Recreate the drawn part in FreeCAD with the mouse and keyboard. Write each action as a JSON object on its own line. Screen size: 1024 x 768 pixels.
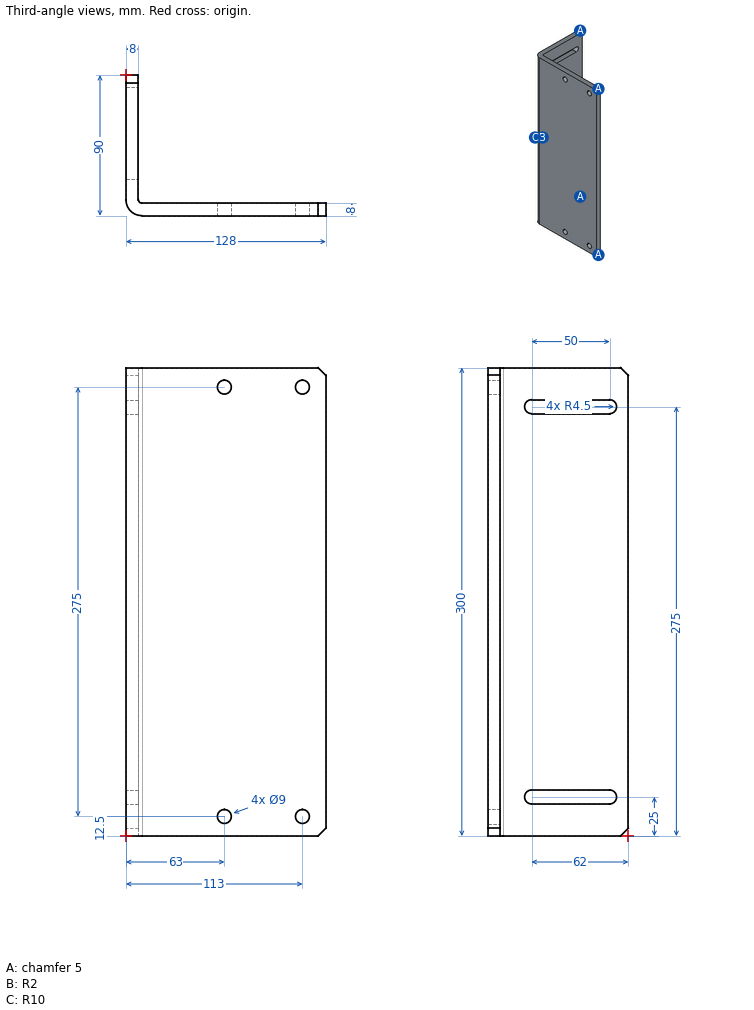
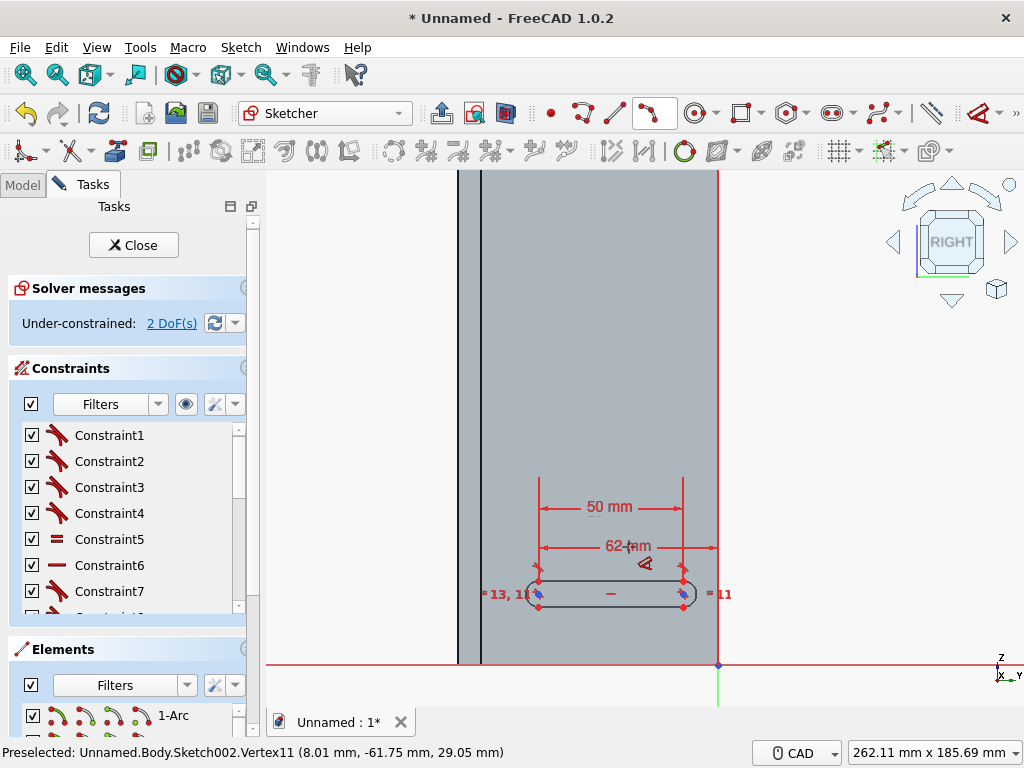
{"action": "left_click", "coordinate": [539, 594]}
{"action": "left_click", "coordinate": [752, 630]}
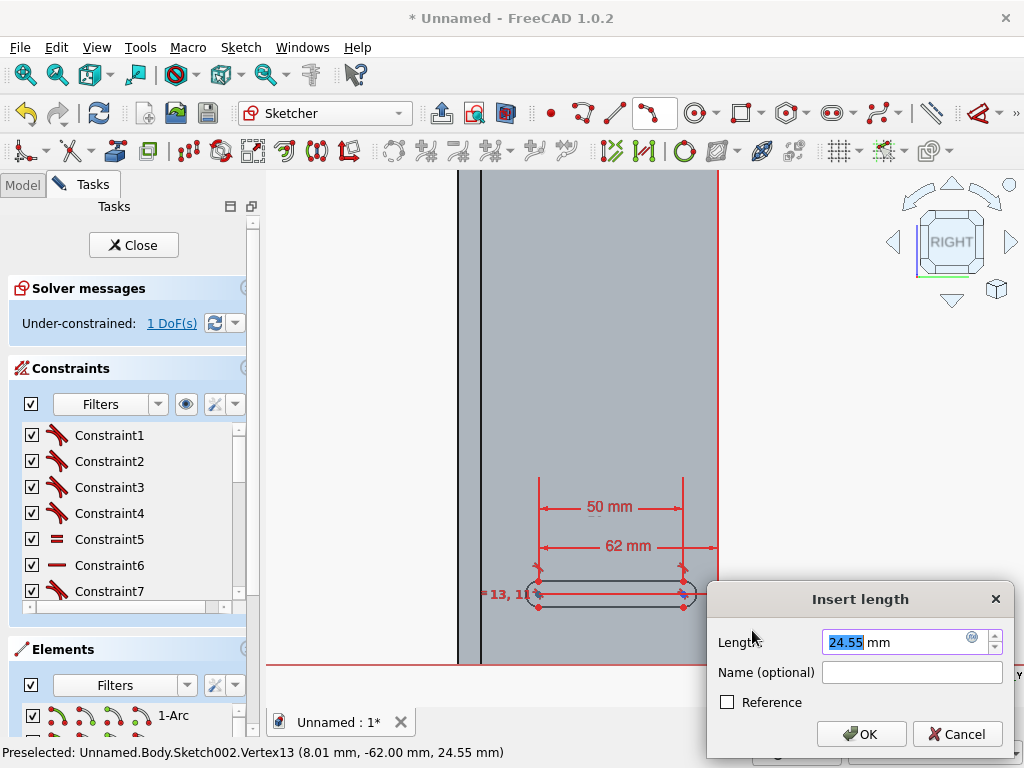
{"action": "type", "text": "25"}
{"action": "key", "text": "Return"}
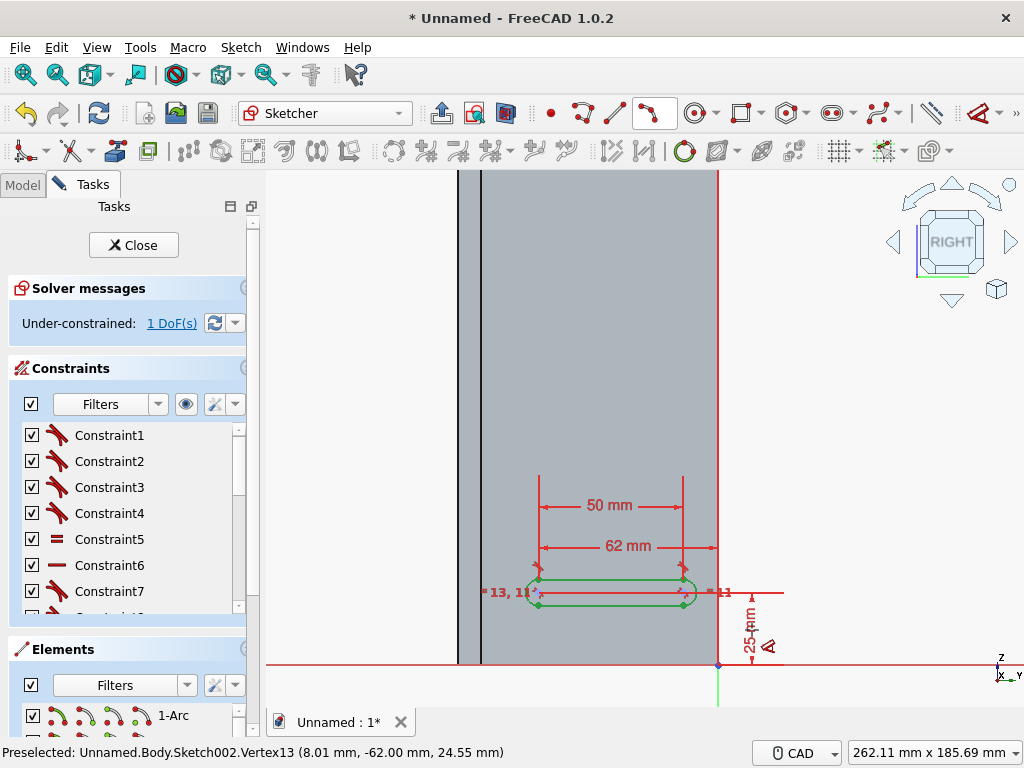
{"action": "scroll", "coordinate": [539, 583], "scroll_direction": "down", "scroll_amount": 4}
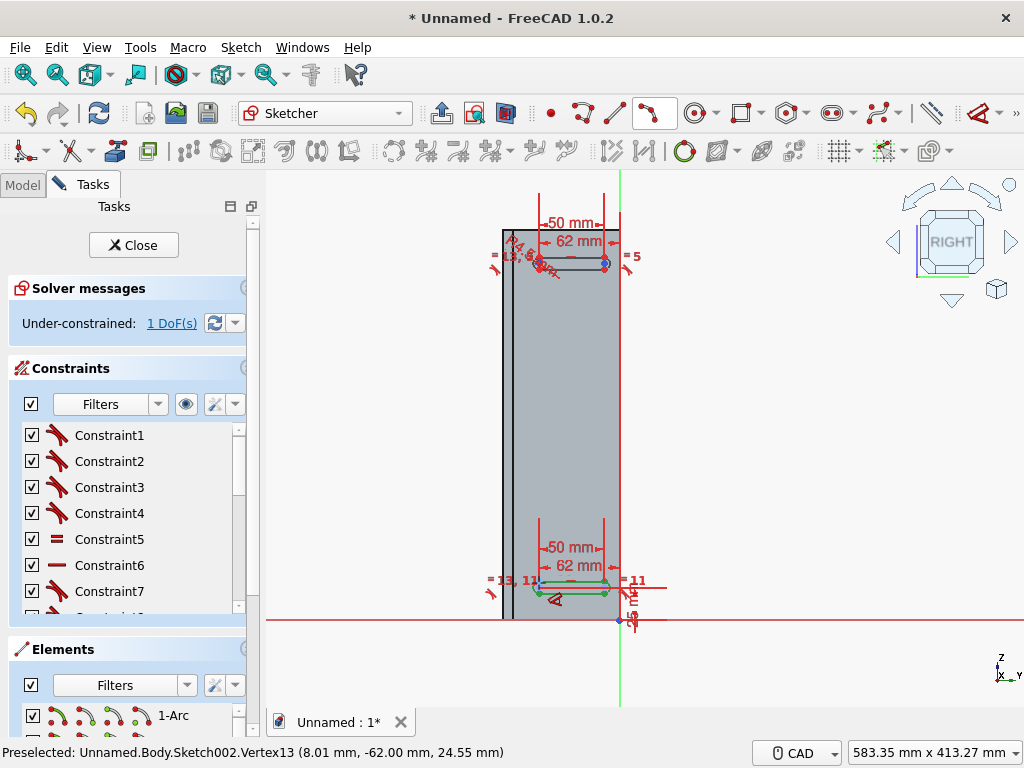
{"action": "scroll", "coordinate": [539, 264], "scroll_direction": "up", "scroll_amount": 4}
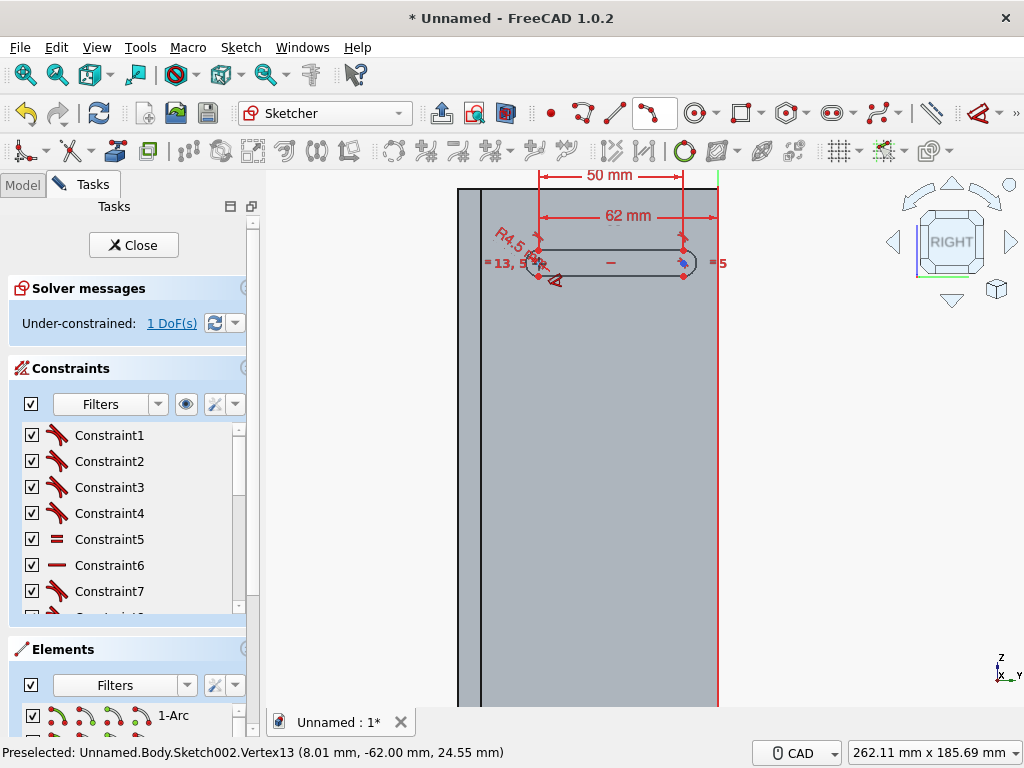
{"action": "left_click", "coordinate": [539, 263]}
{"action": "left_click", "coordinate": [752, 471]}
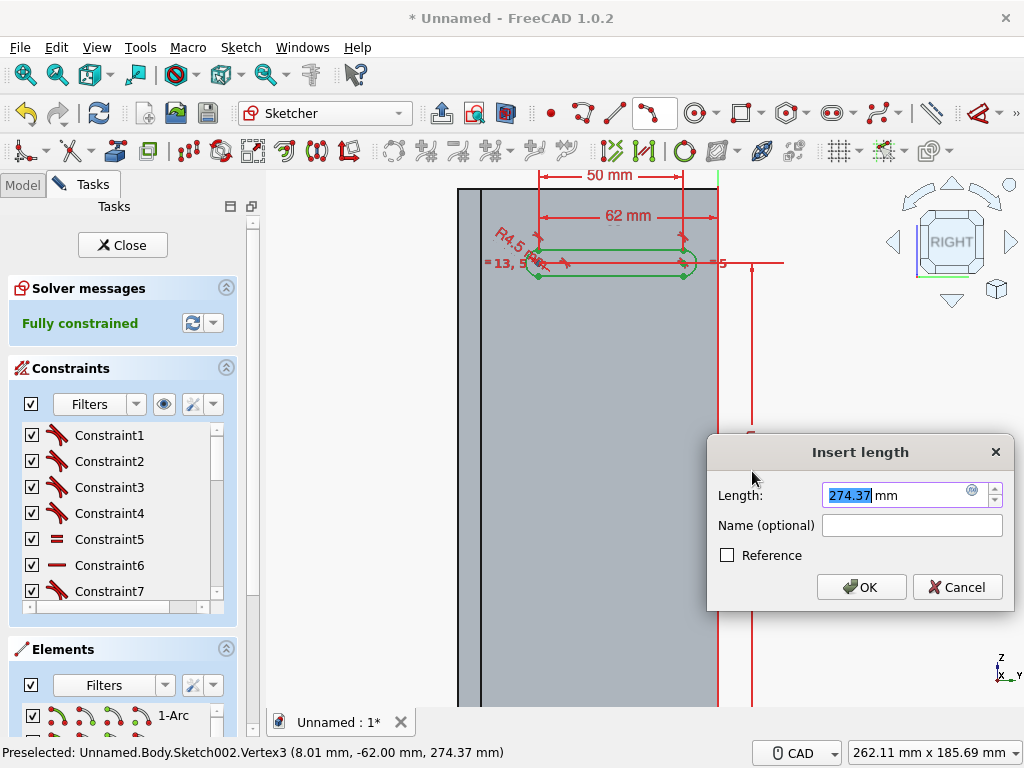
{"action": "type", "text": "275"}
{"action": "key", "text": "Return"}
{"action": "key", "text": "Escape"}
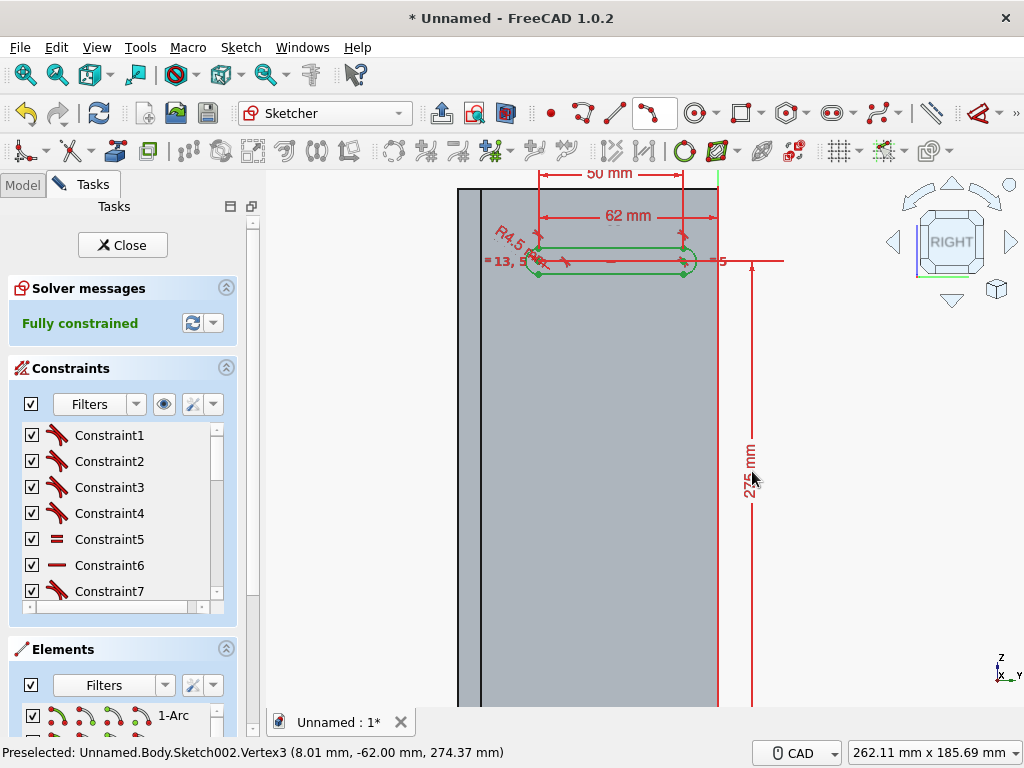
{"action": "left_click", "coordinate": [123, 245]}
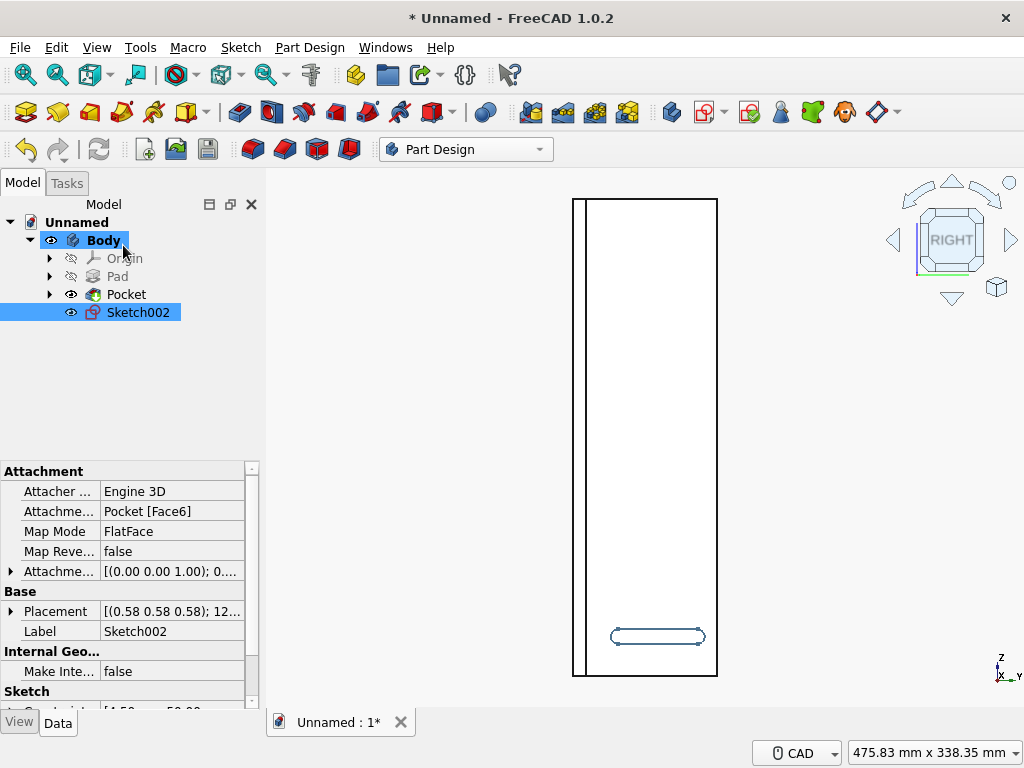
{"action": "left_click", "coordinate": [240, 112]}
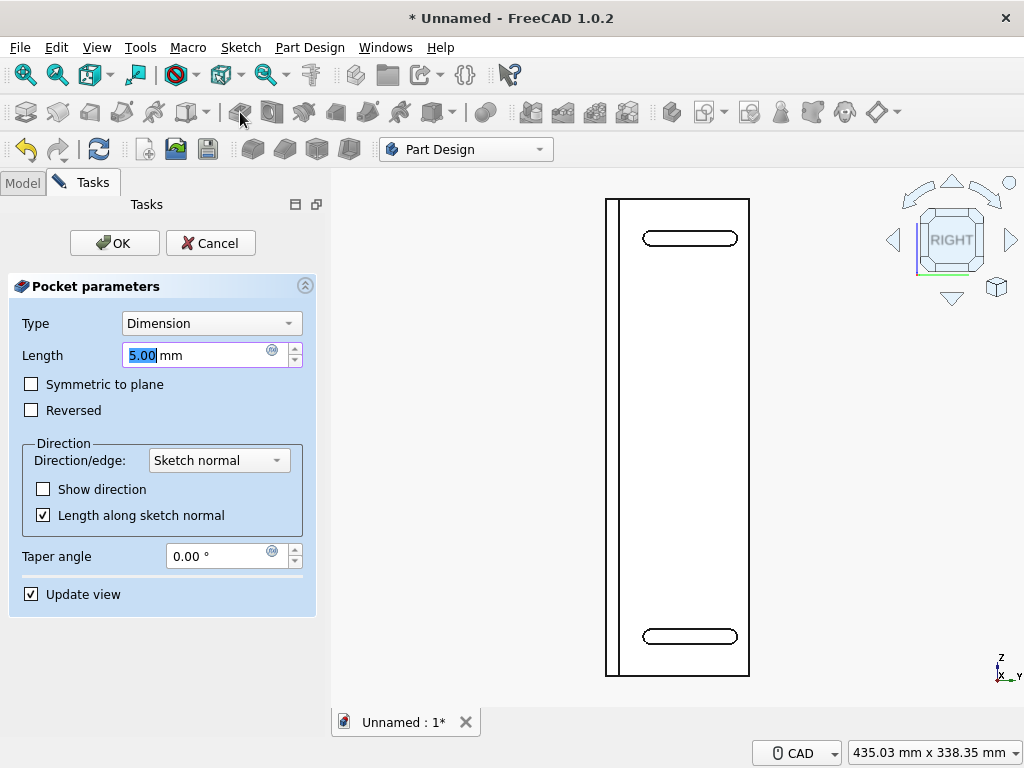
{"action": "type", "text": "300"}
{"action": "key", "text": "Tab"}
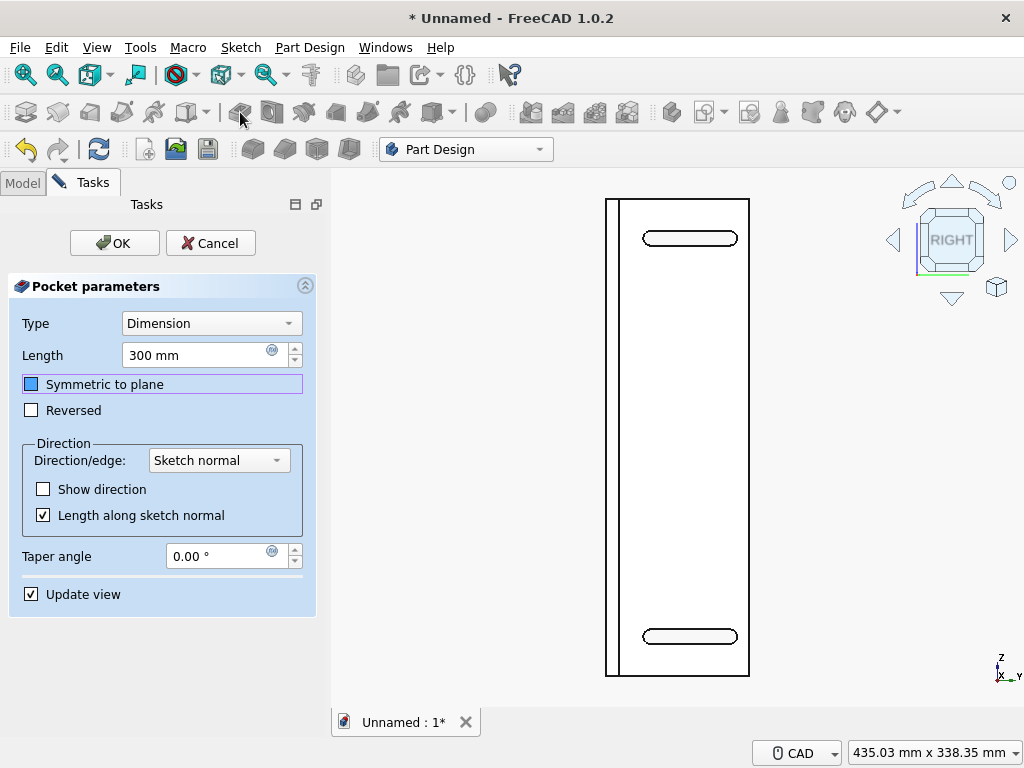
{"action": "left_click", "coordinate": [115, 243]}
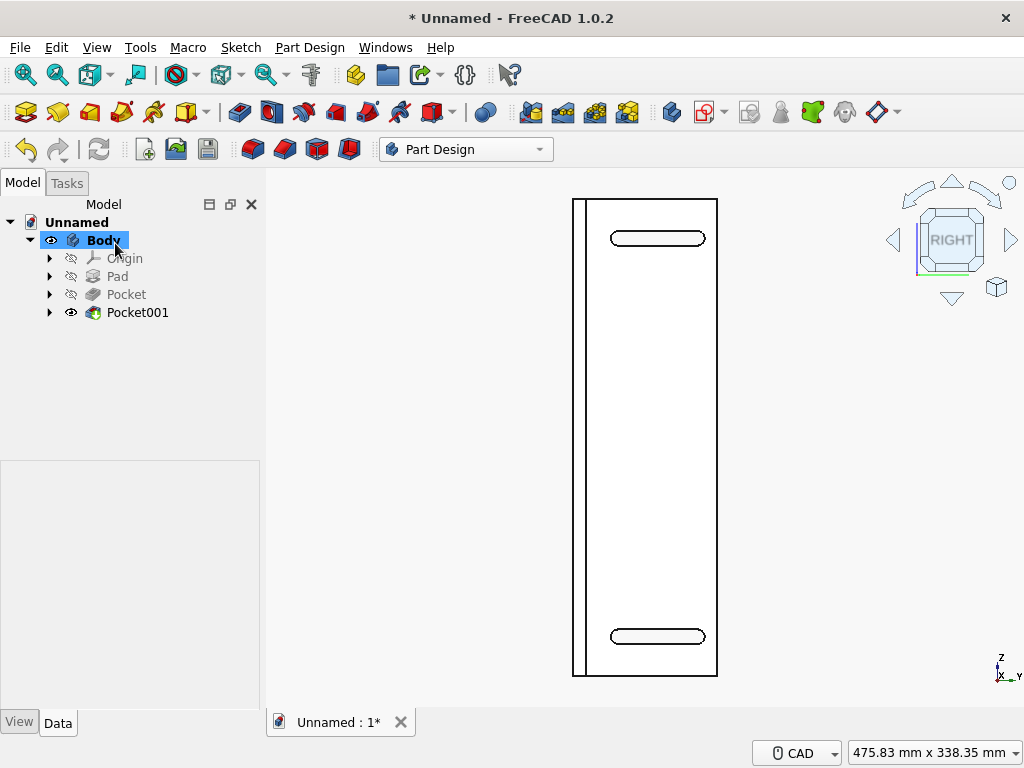
{"action": "left_click", "coordinate": [580, 675]}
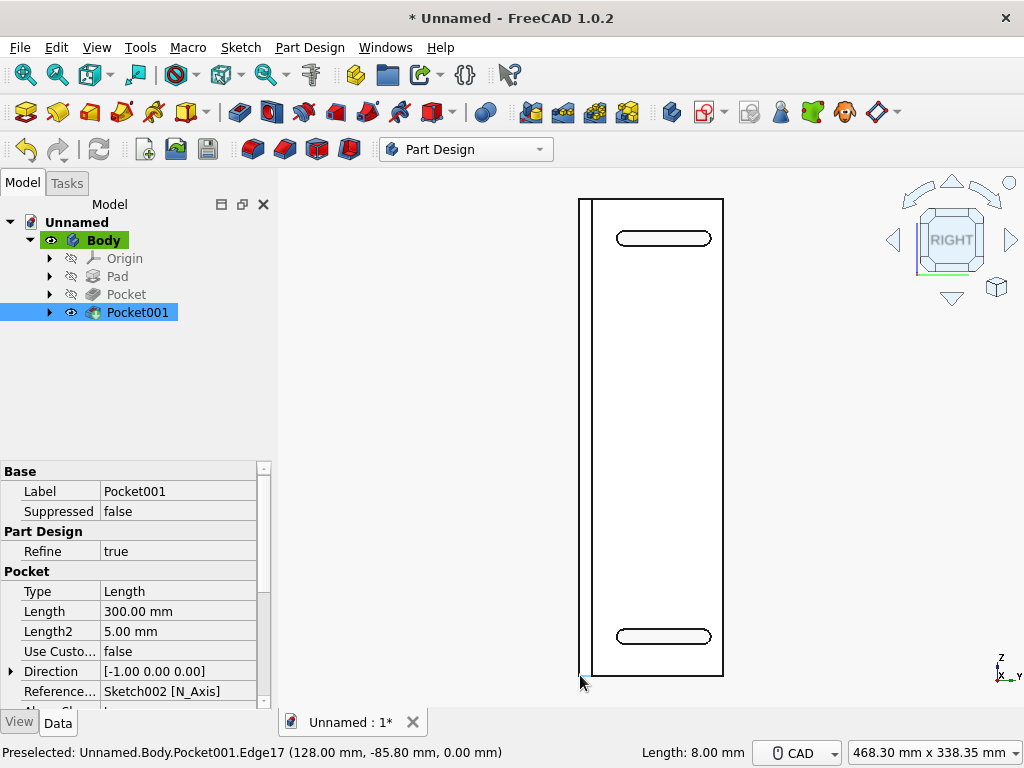
{"action": "scroll", "coordinate": [723, 198], "scroll_direction": "up", "scroll_amount": 6}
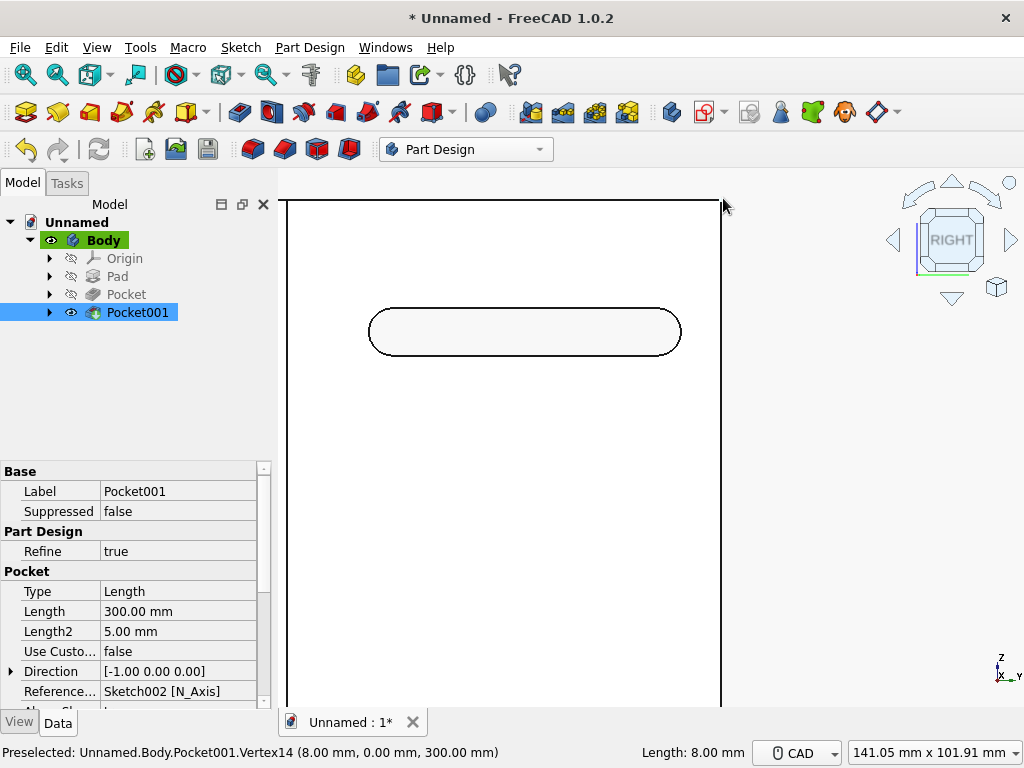
{"action": "left_click", "coordinate": [26, 76]}